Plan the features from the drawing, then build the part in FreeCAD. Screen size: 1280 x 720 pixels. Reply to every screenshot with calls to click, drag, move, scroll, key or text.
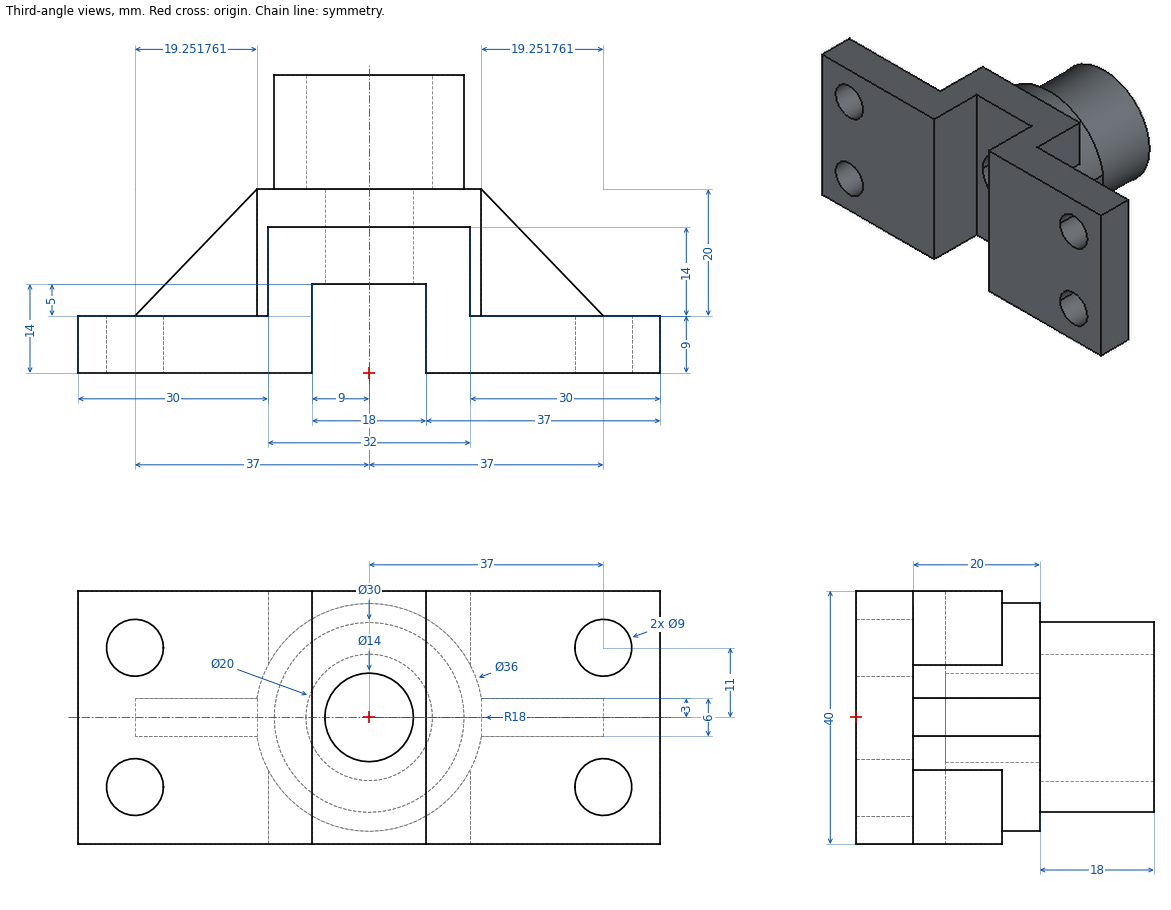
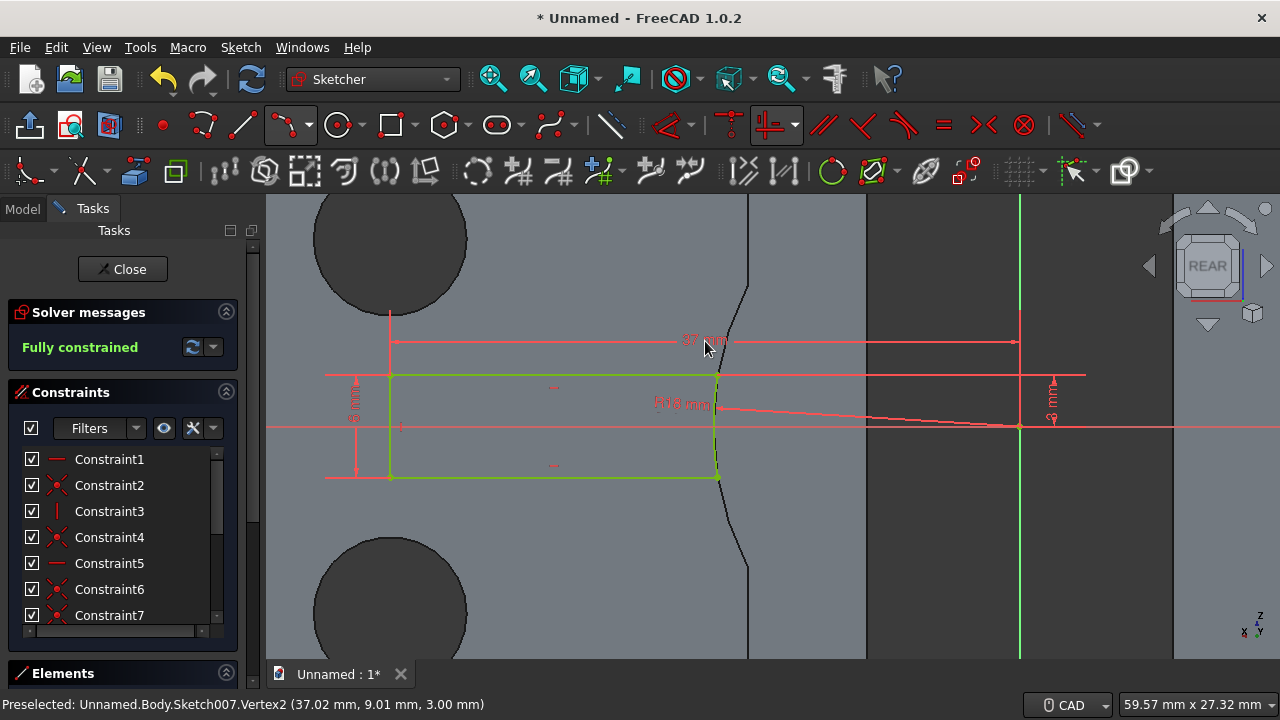
click(123, 269)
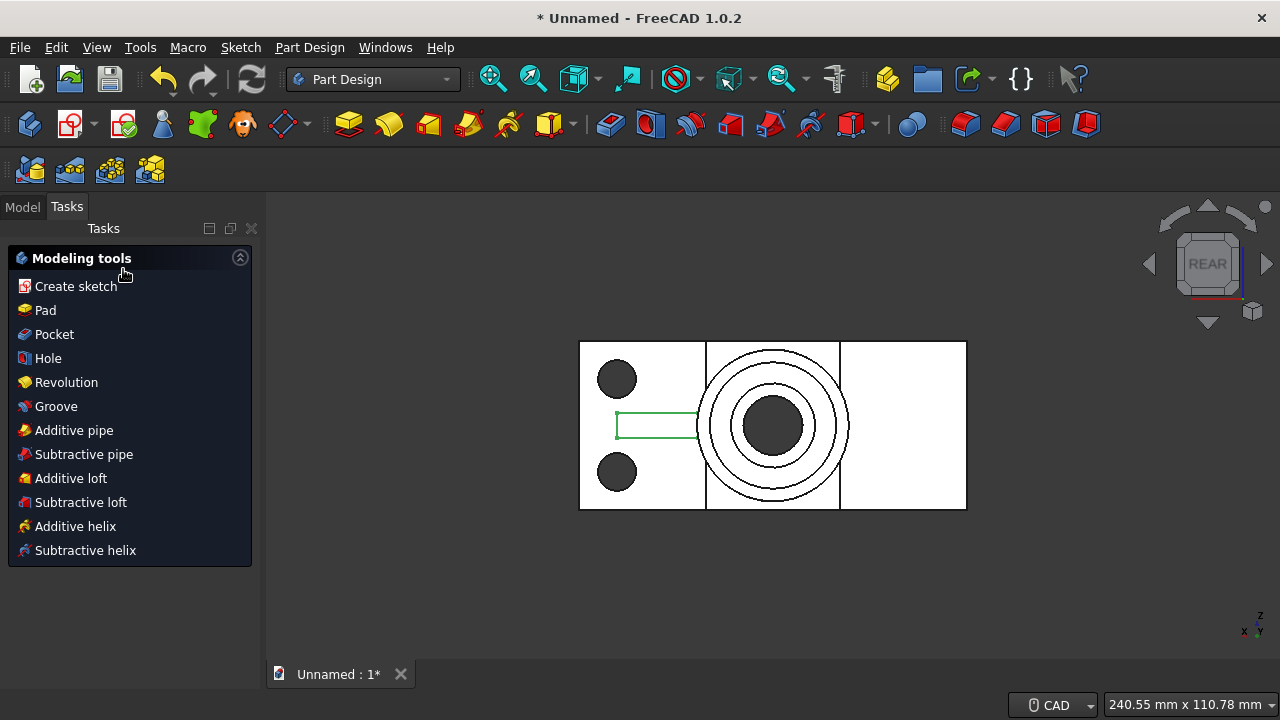
click(350, 124)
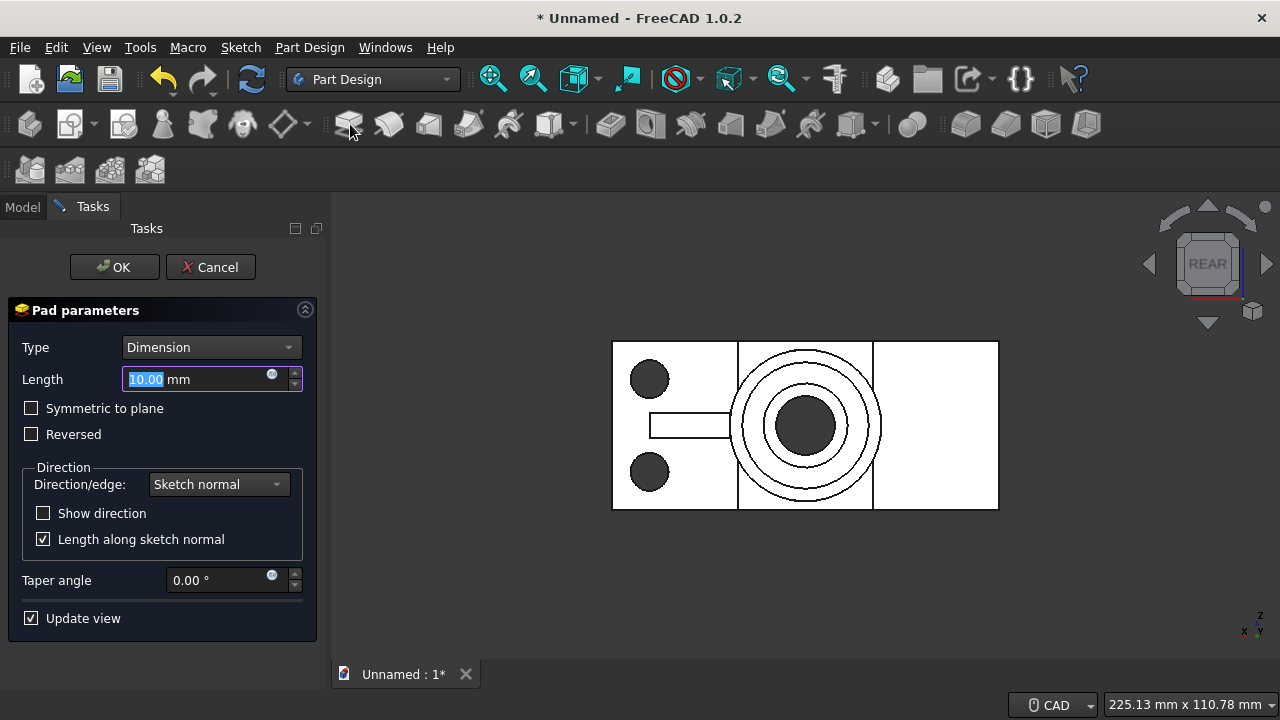
text(20)
key(Tab)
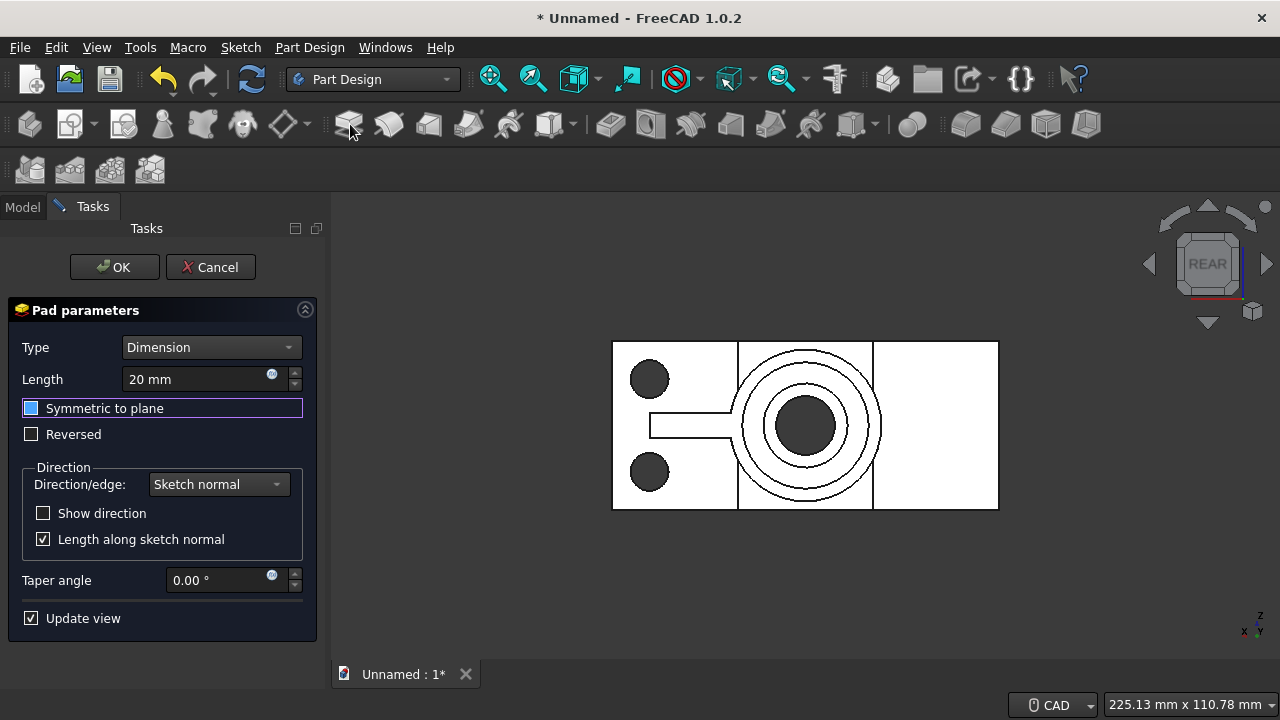
click(115, 267)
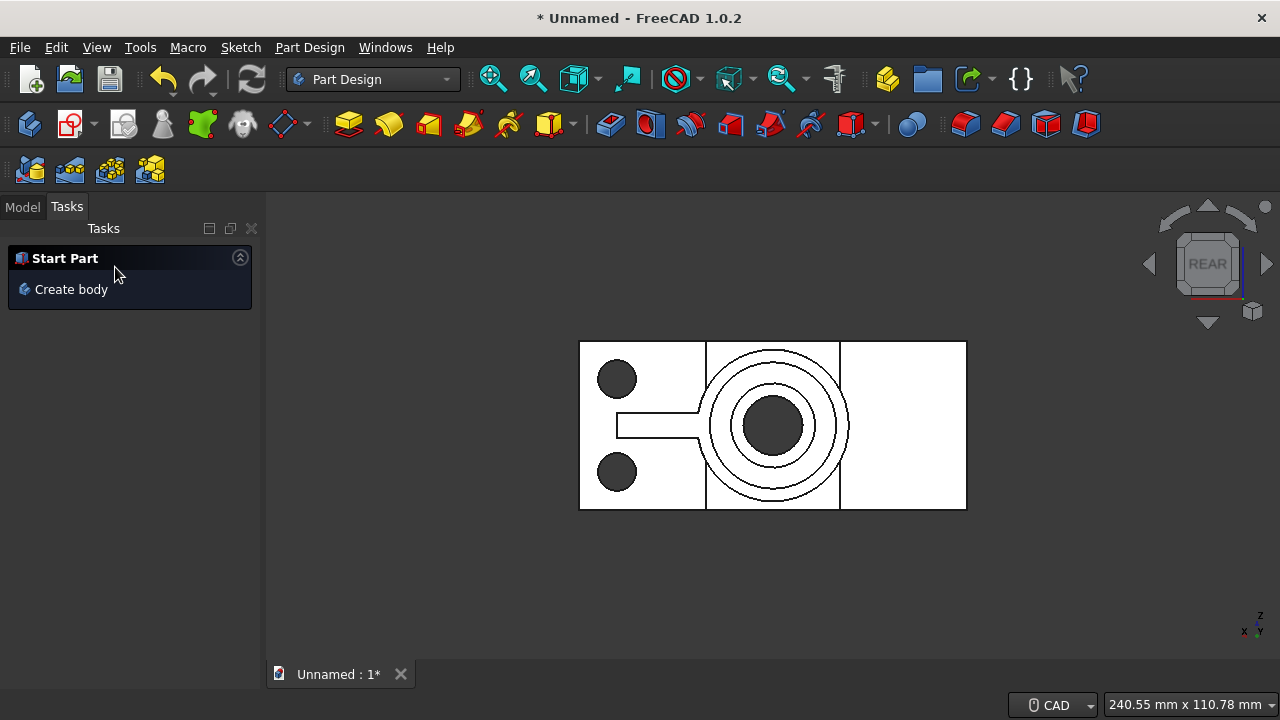
key(v)
key(f)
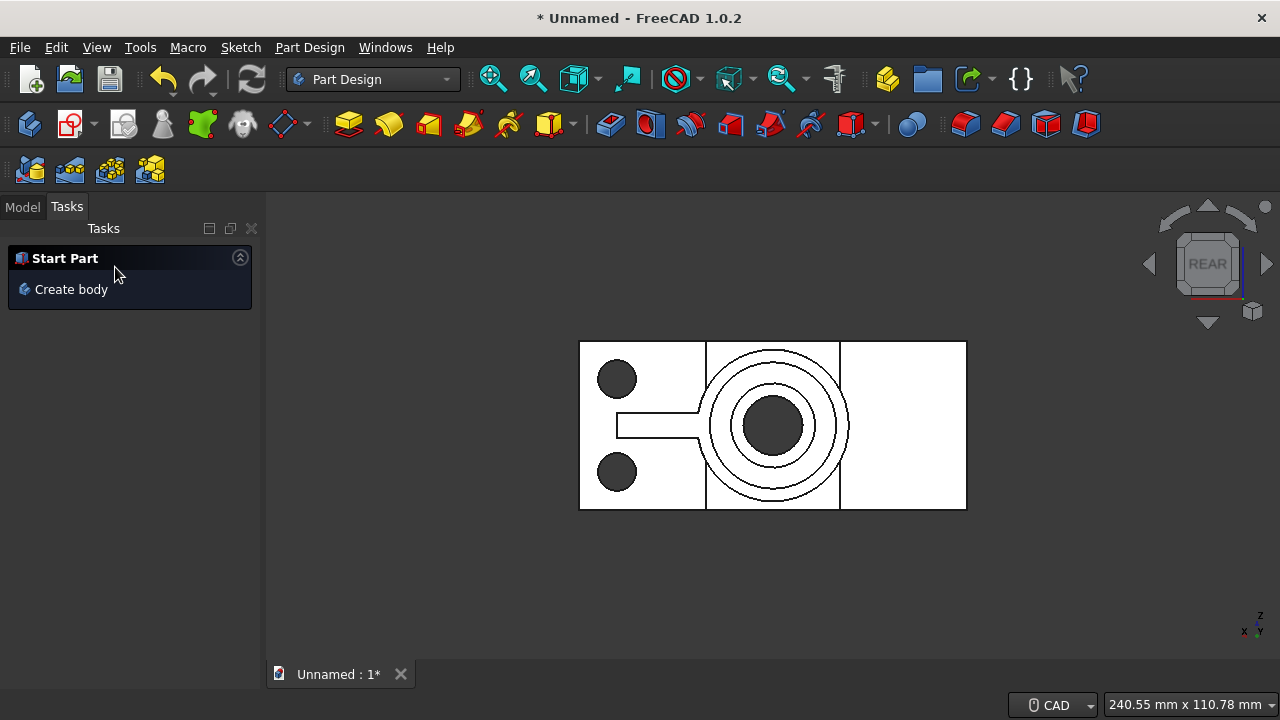
key(0)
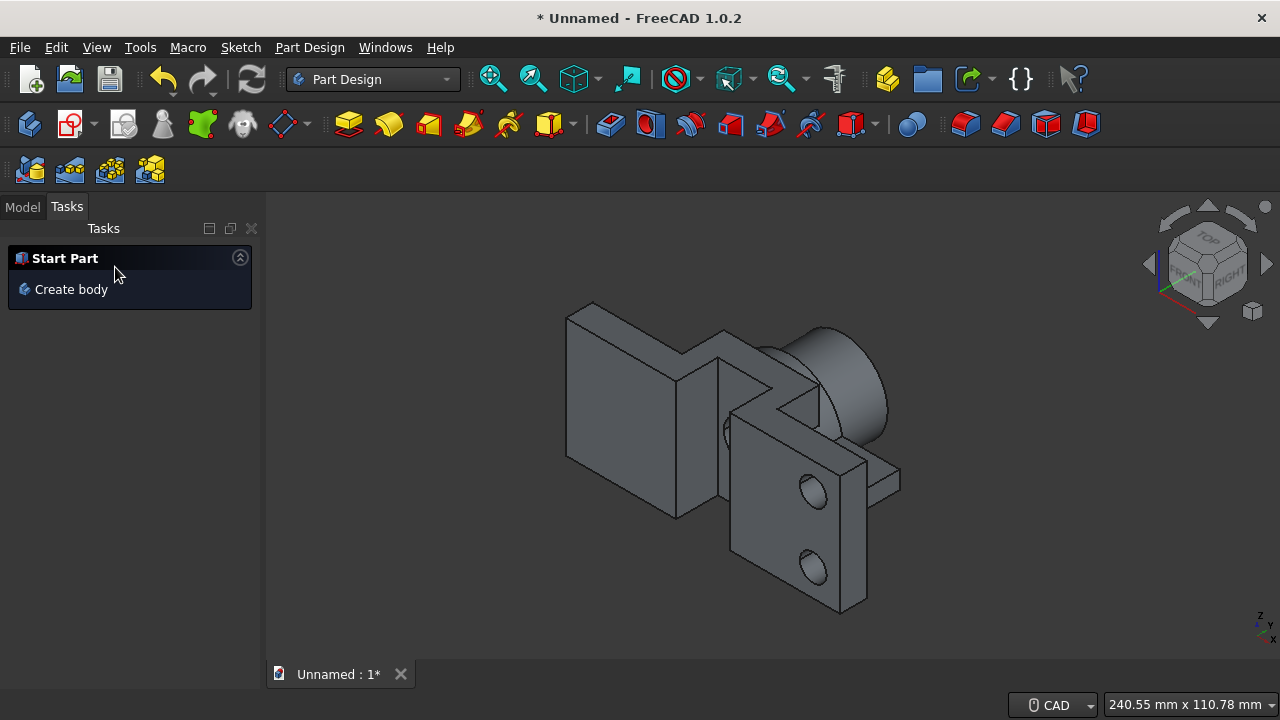
key(2)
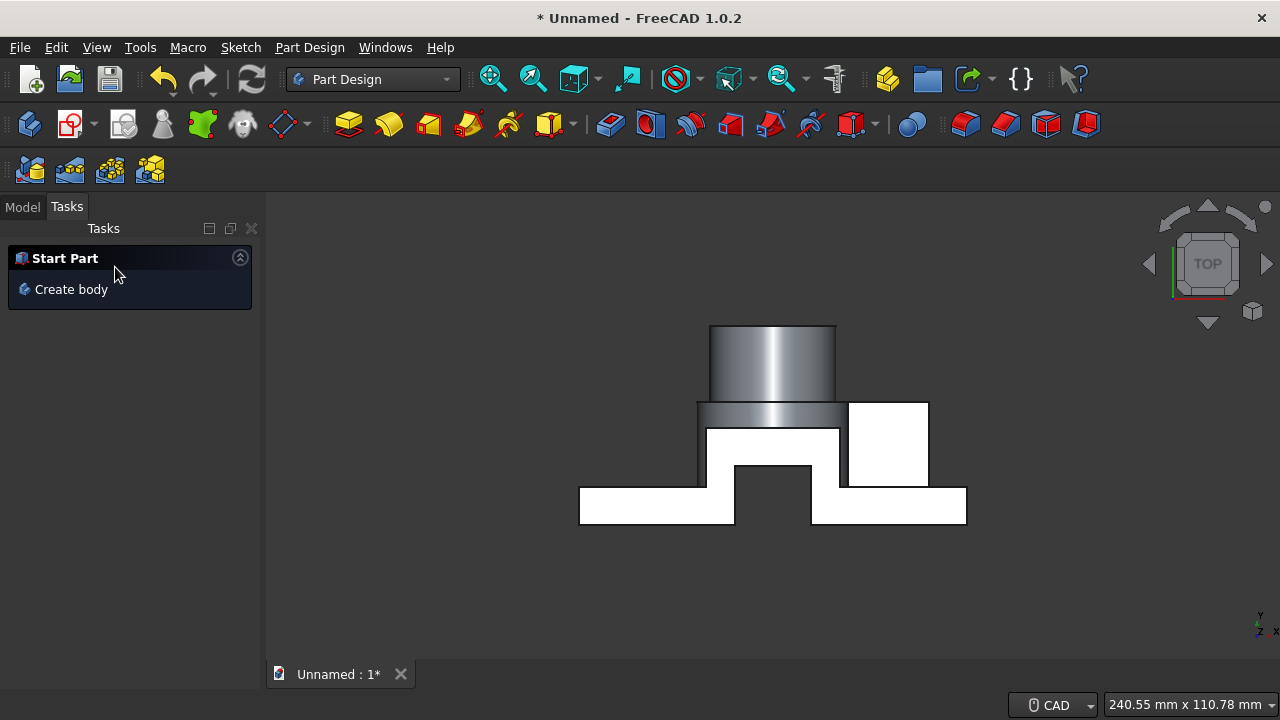
key(v)
key(f)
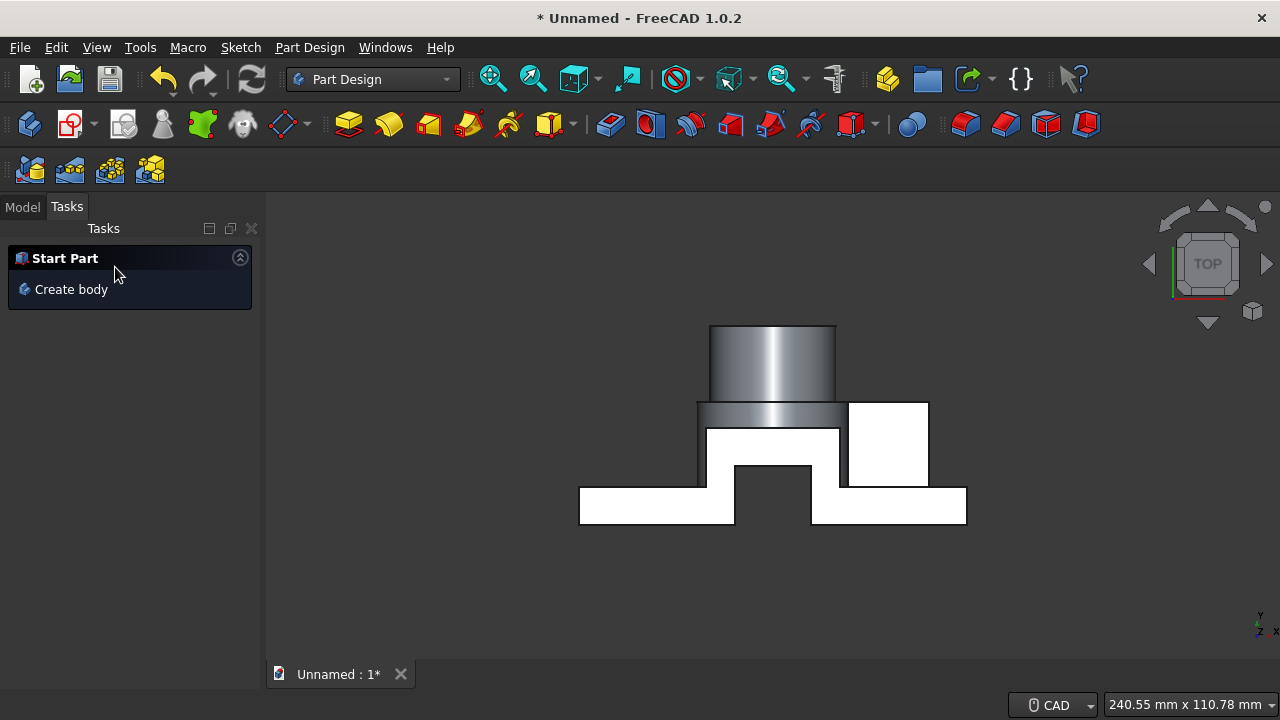
click(888, 443)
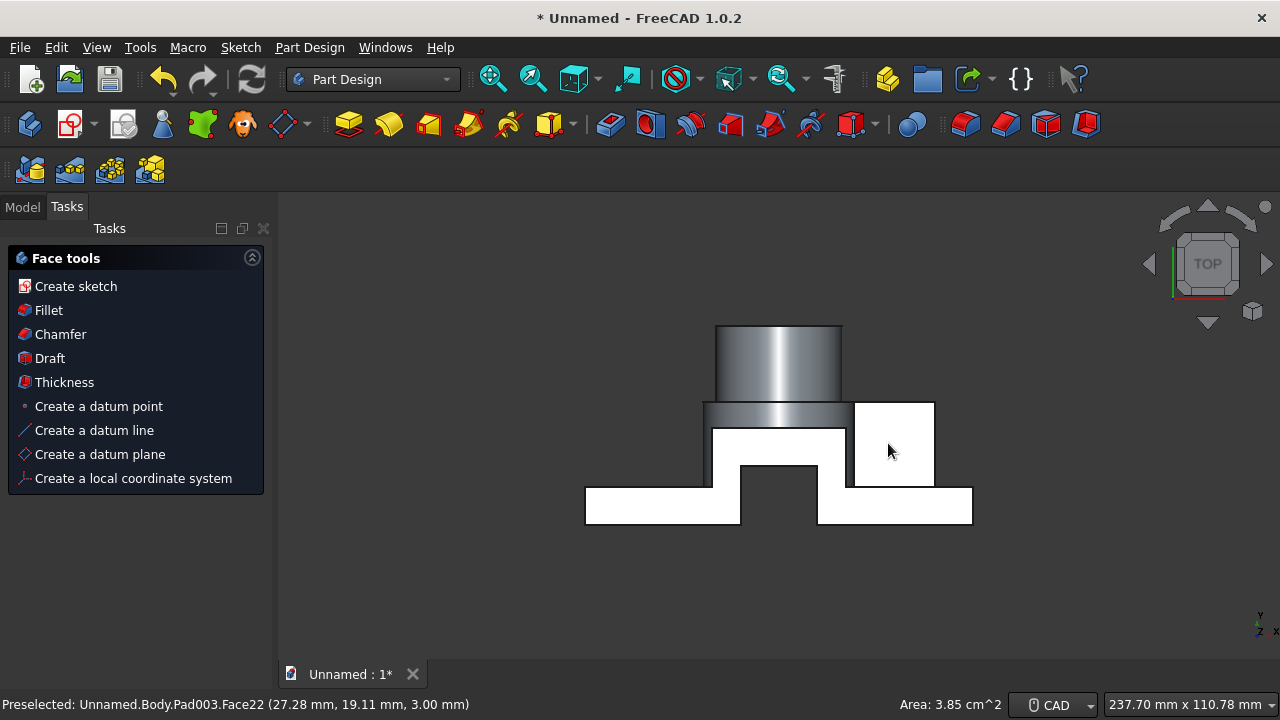
click(70, 124)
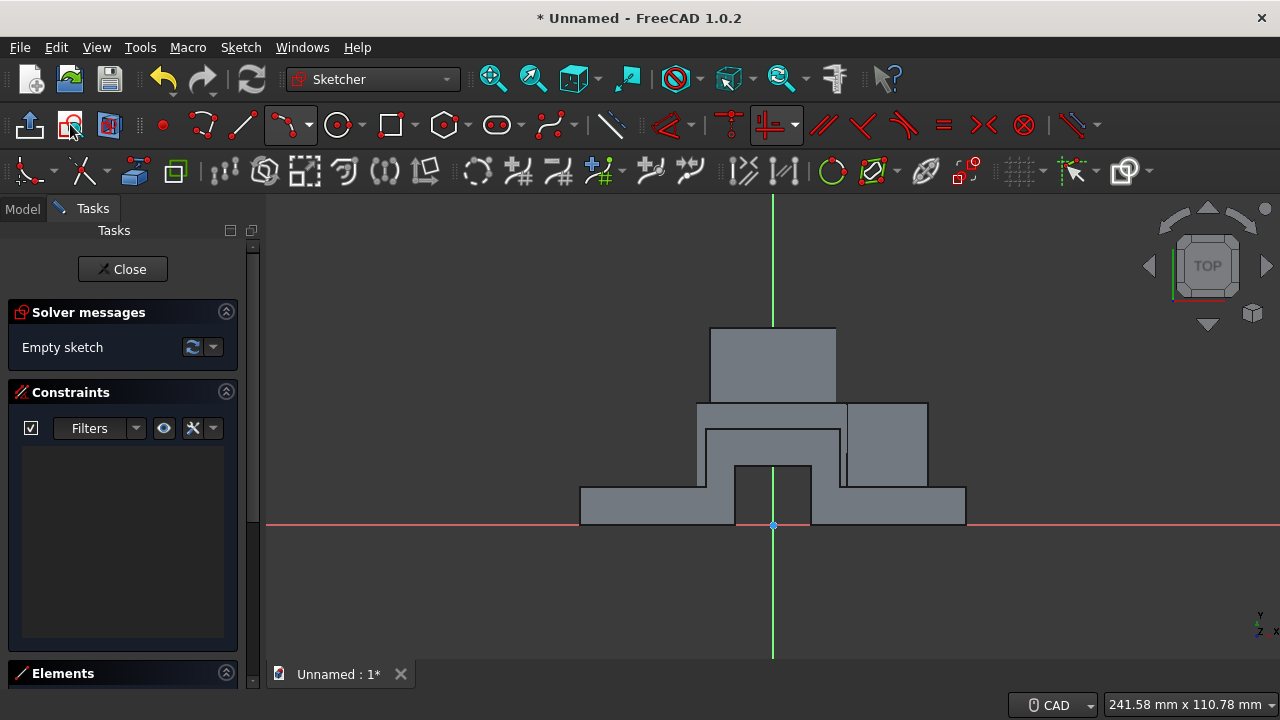
scroll(970, 495, up, 4)